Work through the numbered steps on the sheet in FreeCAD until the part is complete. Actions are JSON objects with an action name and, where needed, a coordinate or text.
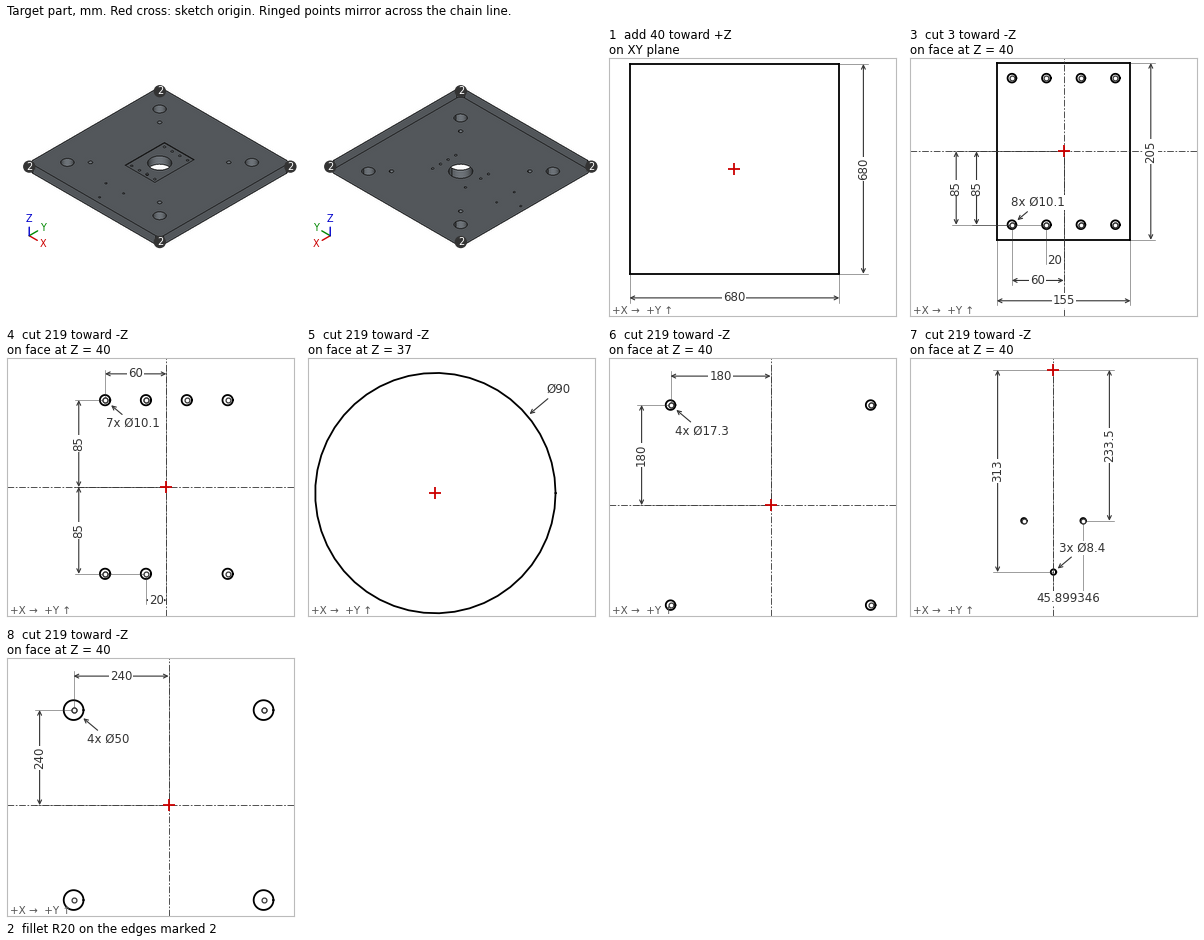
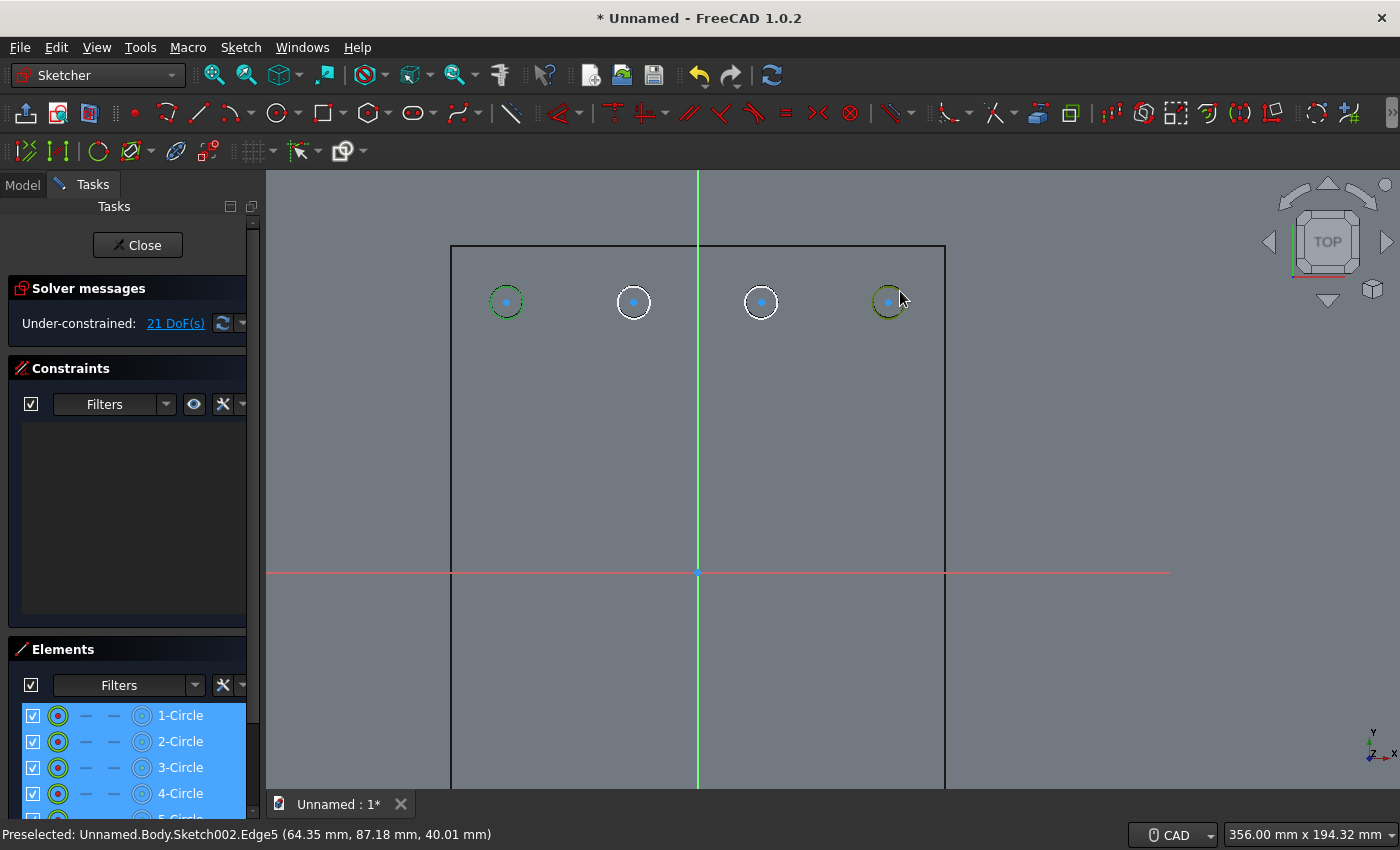
{"action": "left_click", "coordinate": [773, 291]}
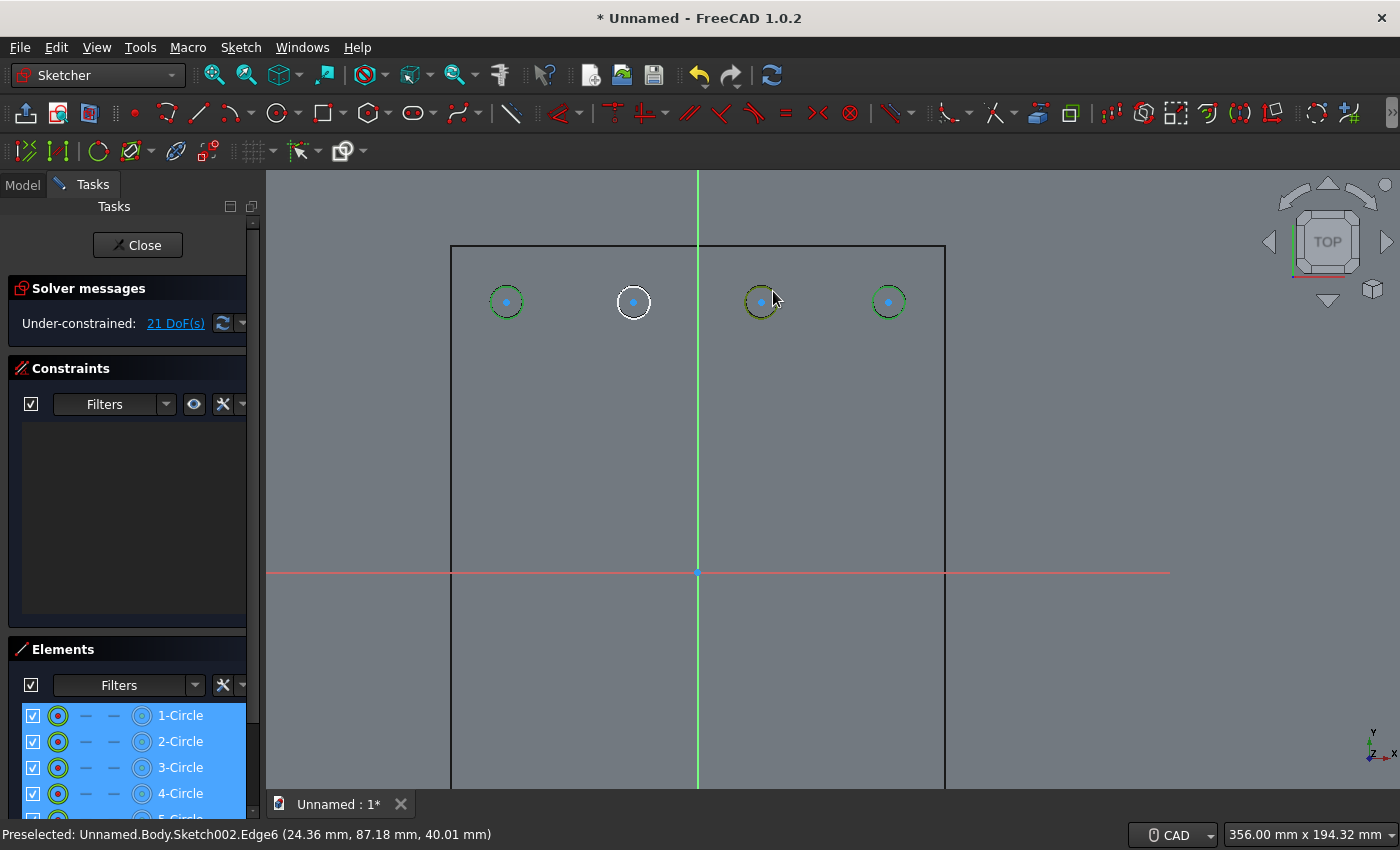
{"action": "left_click", "coordinate": [645, 291]}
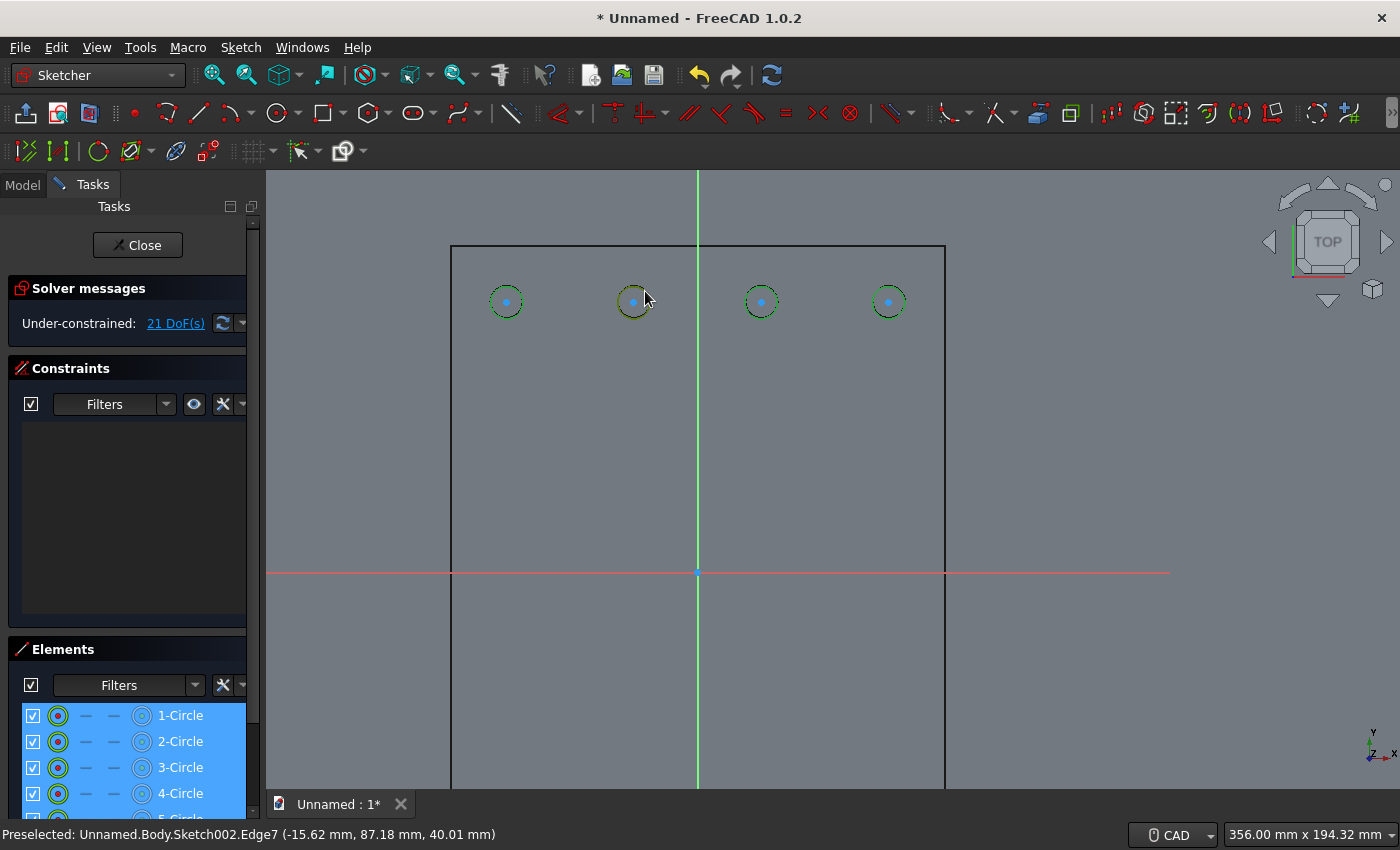
{"action": "left_click", "coordinate": [786, 114]}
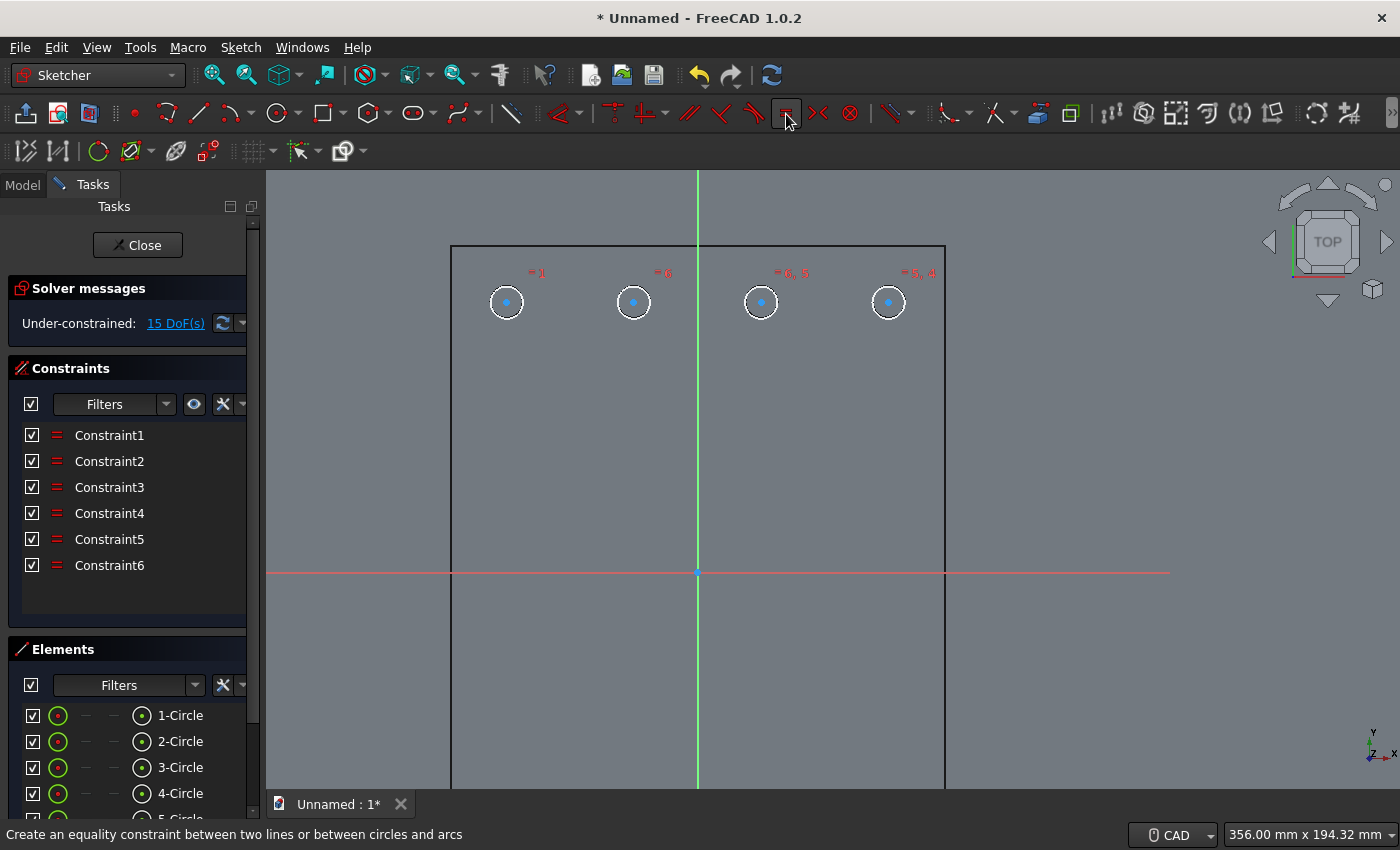
{"action": "left_click", "coordinate": [507, 303]}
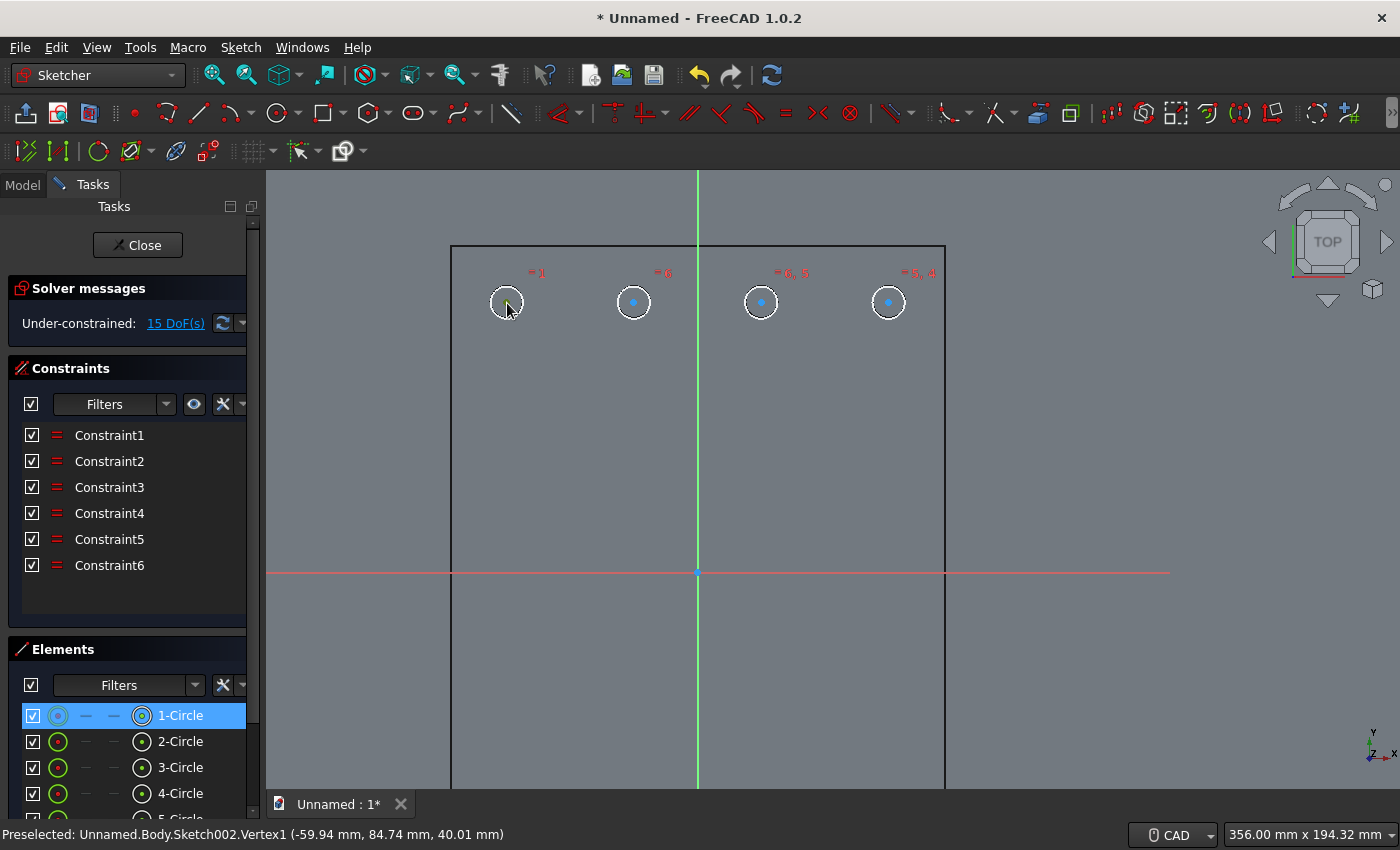
{"action": "scroll", "coordinate": [900, 290], "scroll_direction": "down", "scroll_amount": 2}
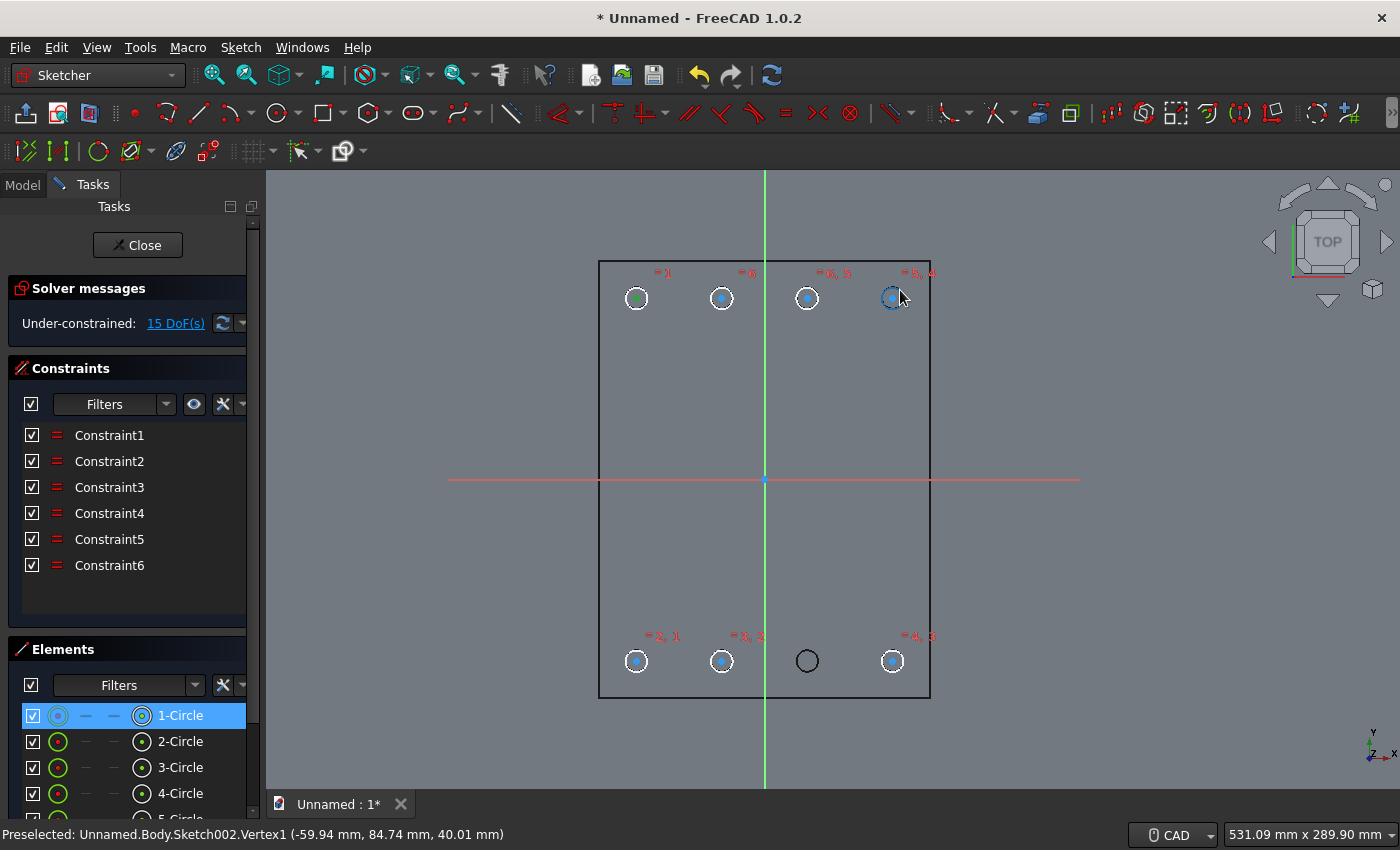
{"action": "left_click", "coordinate": [636, 661]}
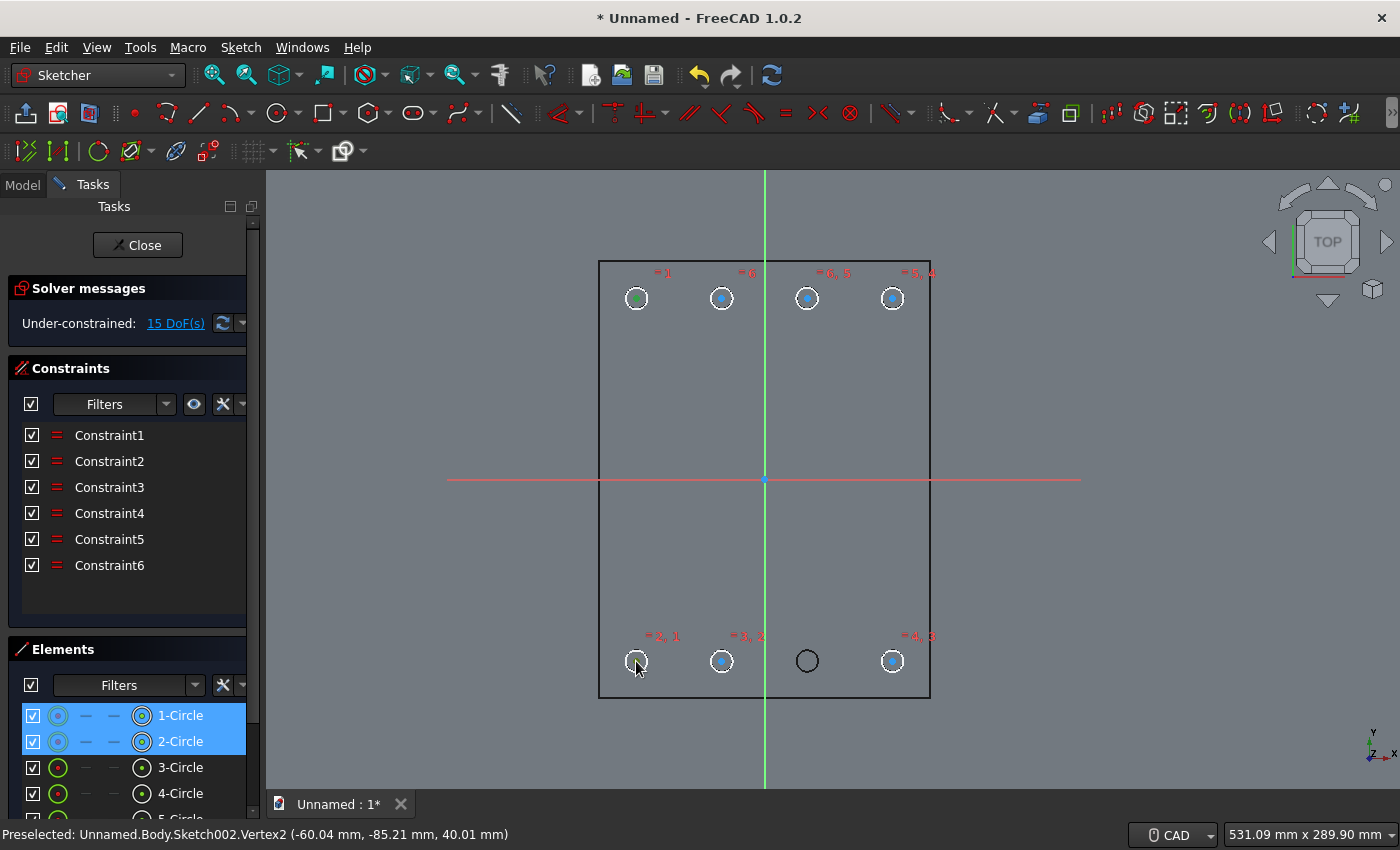
{"action": "left_click", "coordinate": [496, 480]}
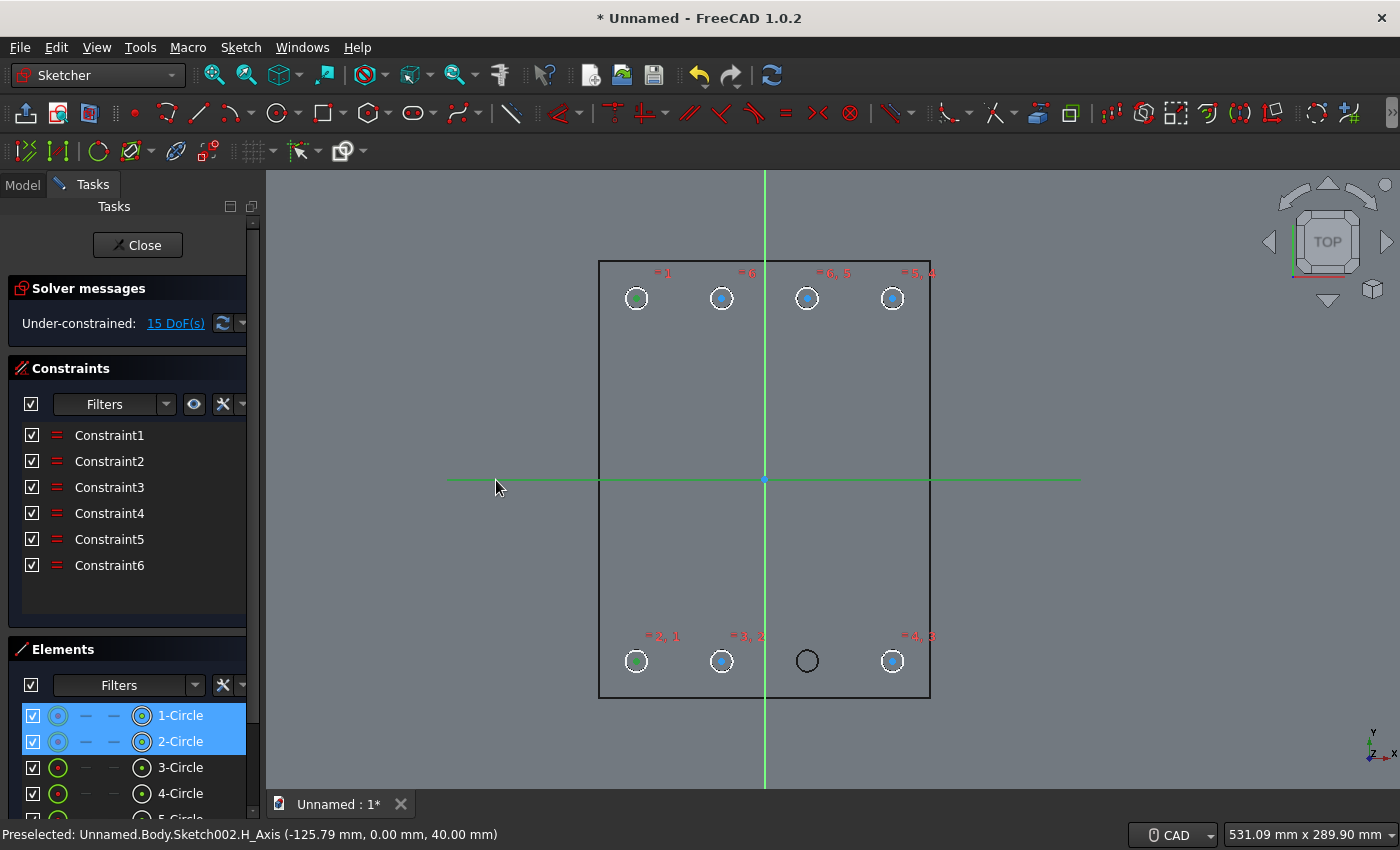
{"action": "left_click", "coordinate": [818, 114]}